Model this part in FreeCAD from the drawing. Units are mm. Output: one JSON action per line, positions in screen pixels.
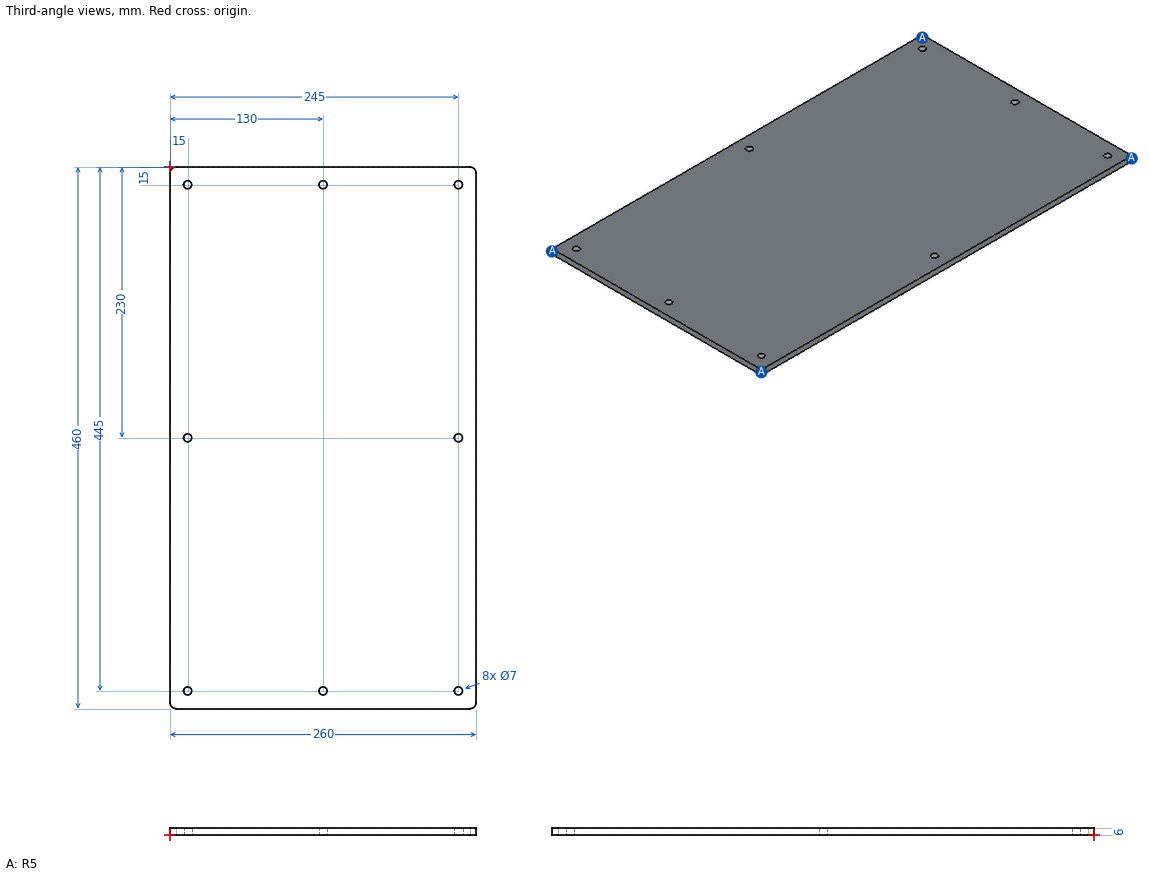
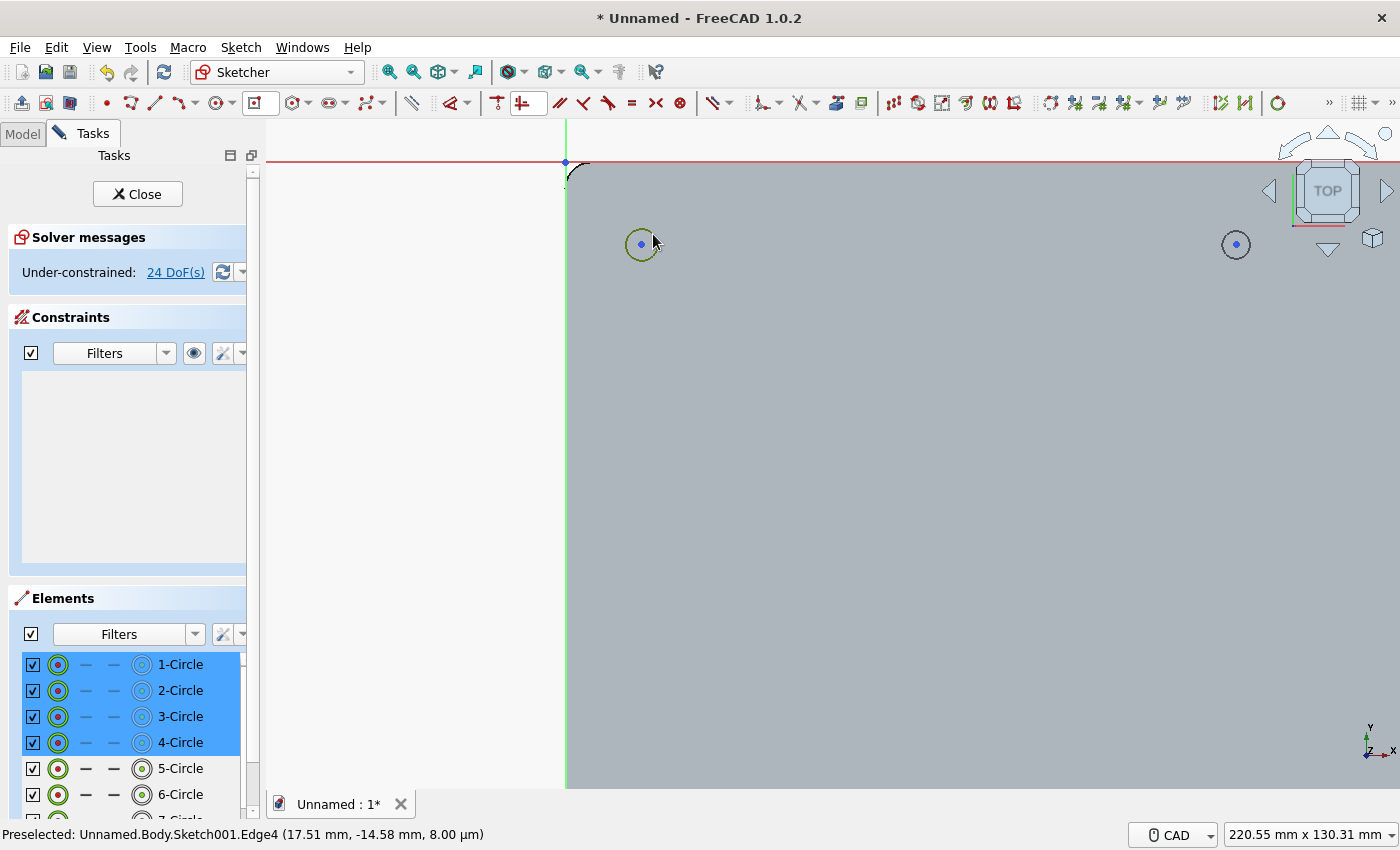
{"action": "scroll", "coordinate": [653, 236], "scroll_direction": "down", "scroll_amount": 8}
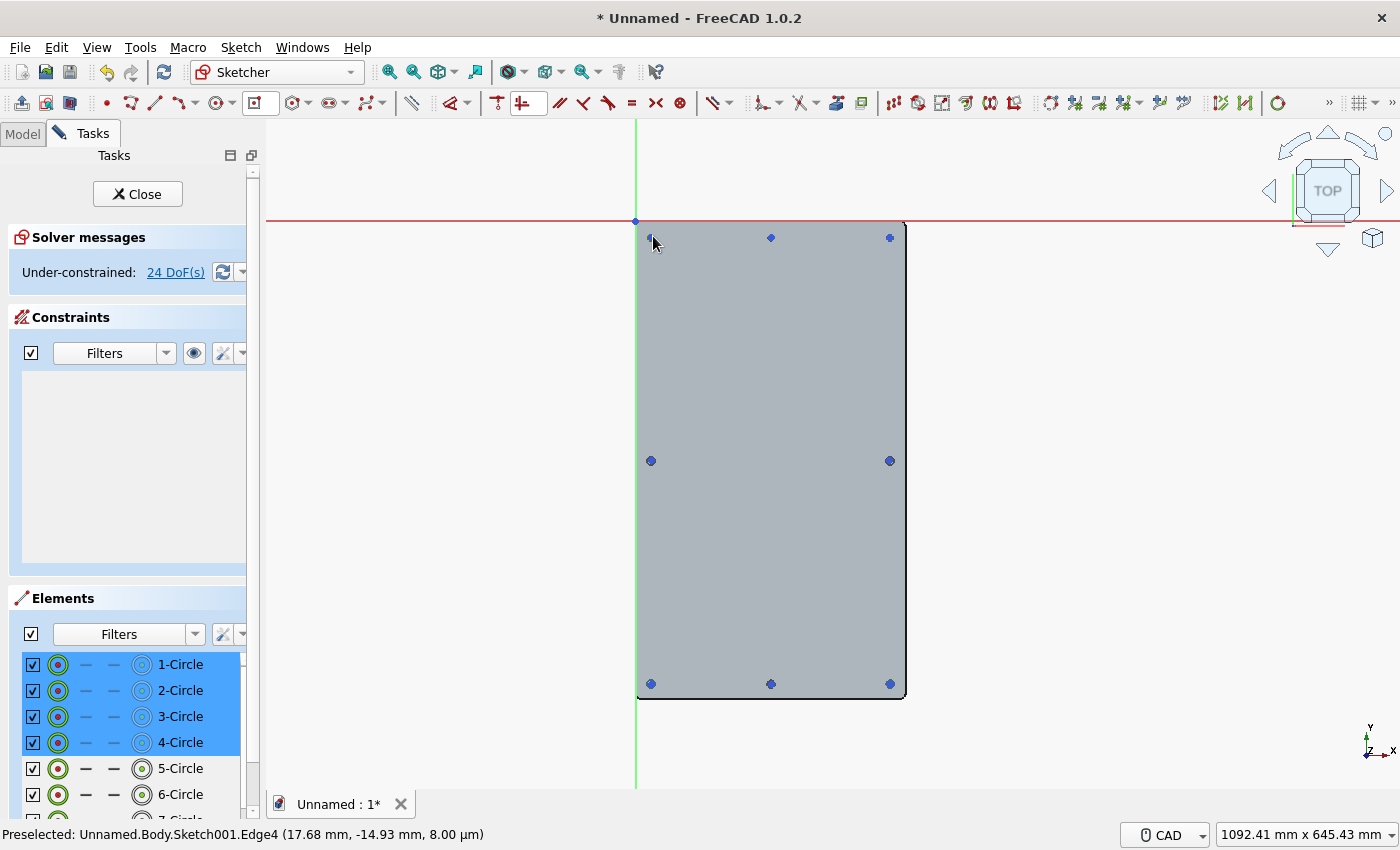
{"action": "scroll", "coordinate": [774, 681], "scroll_direction": "up", "scroll_amount": 7}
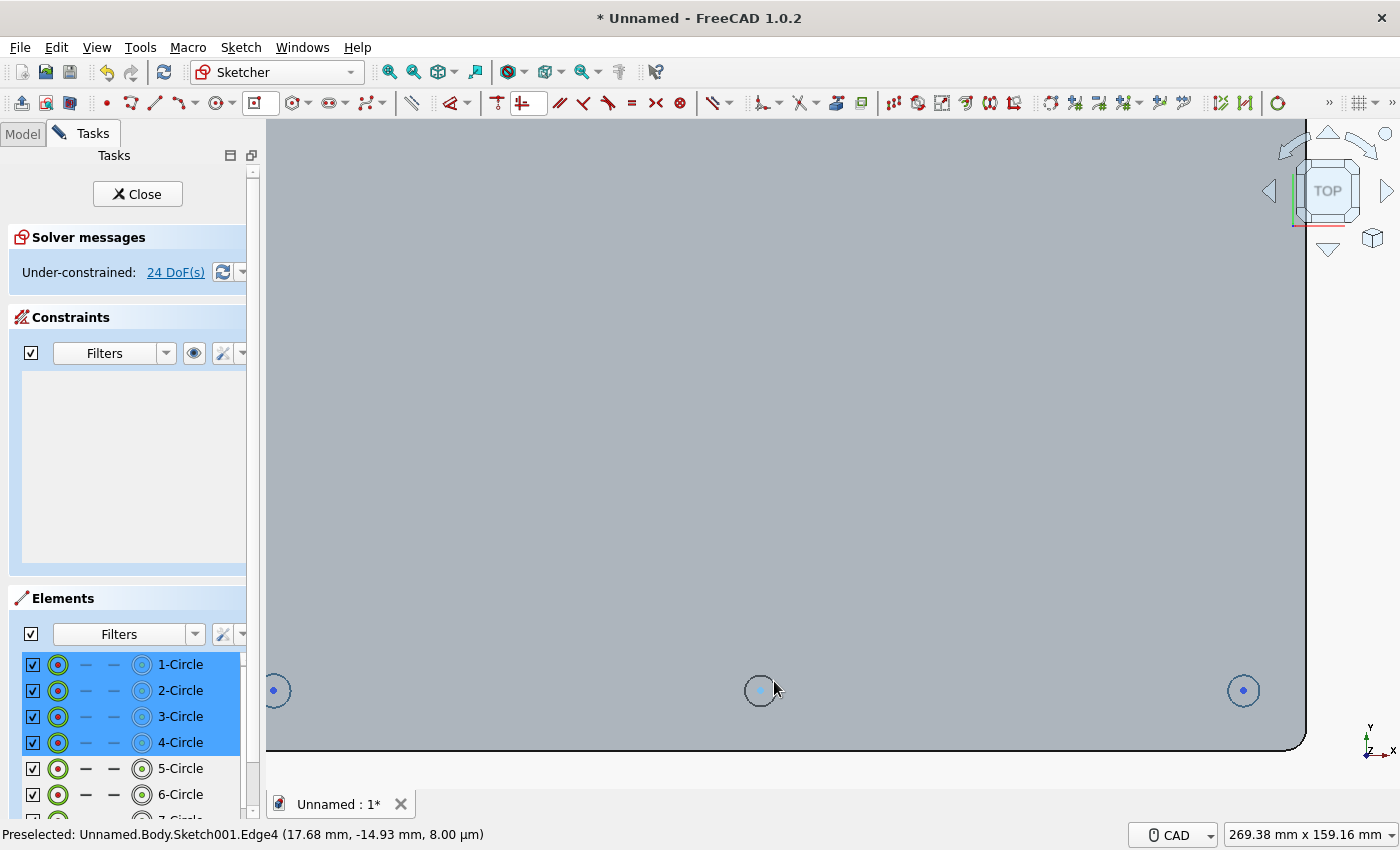
{"action": "left_click", "coordinate": [771, 680]}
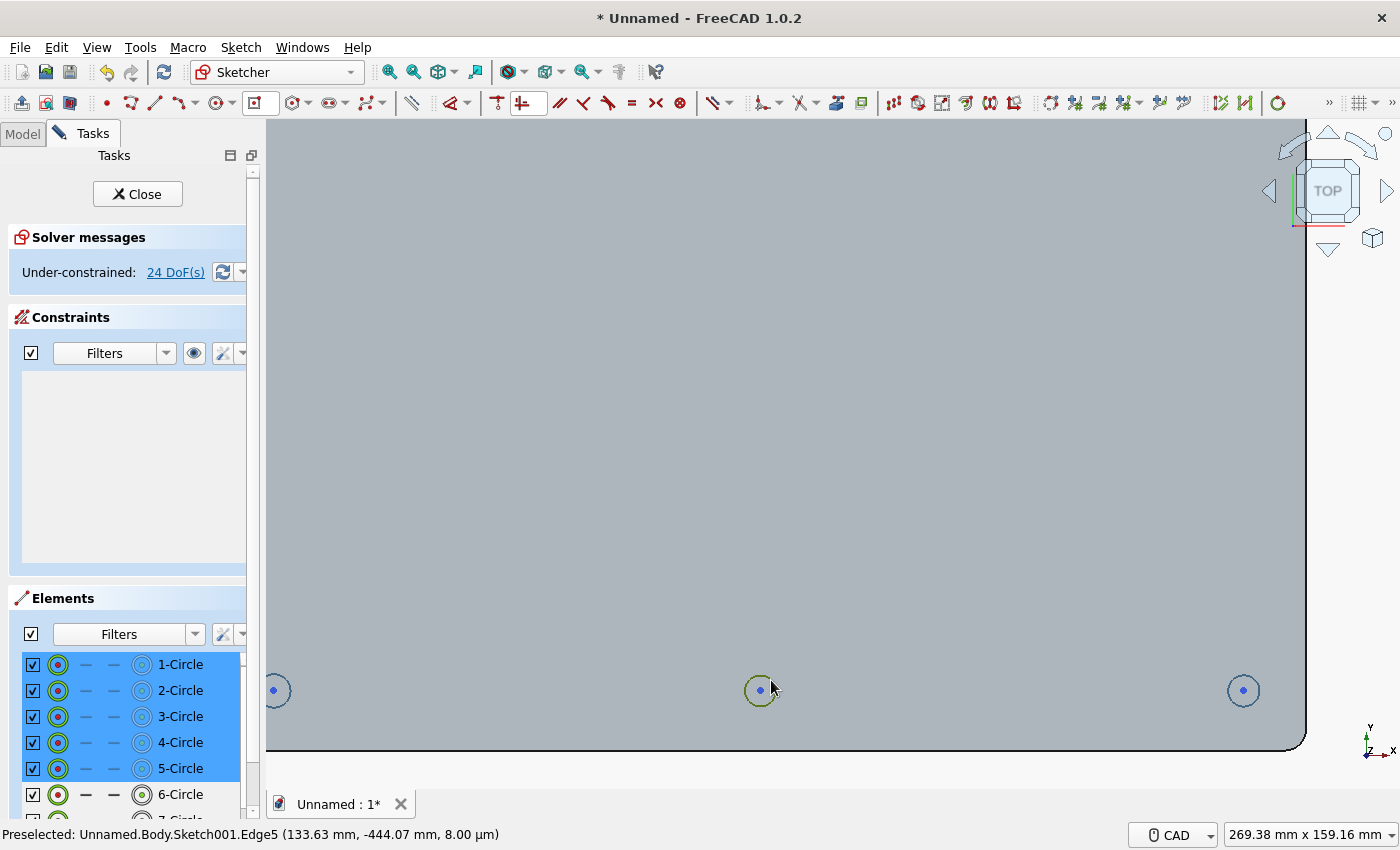
{"action": "scroll", "coordinate": [774, 682], "scroll_direction": "down", "scroll_amount": 7}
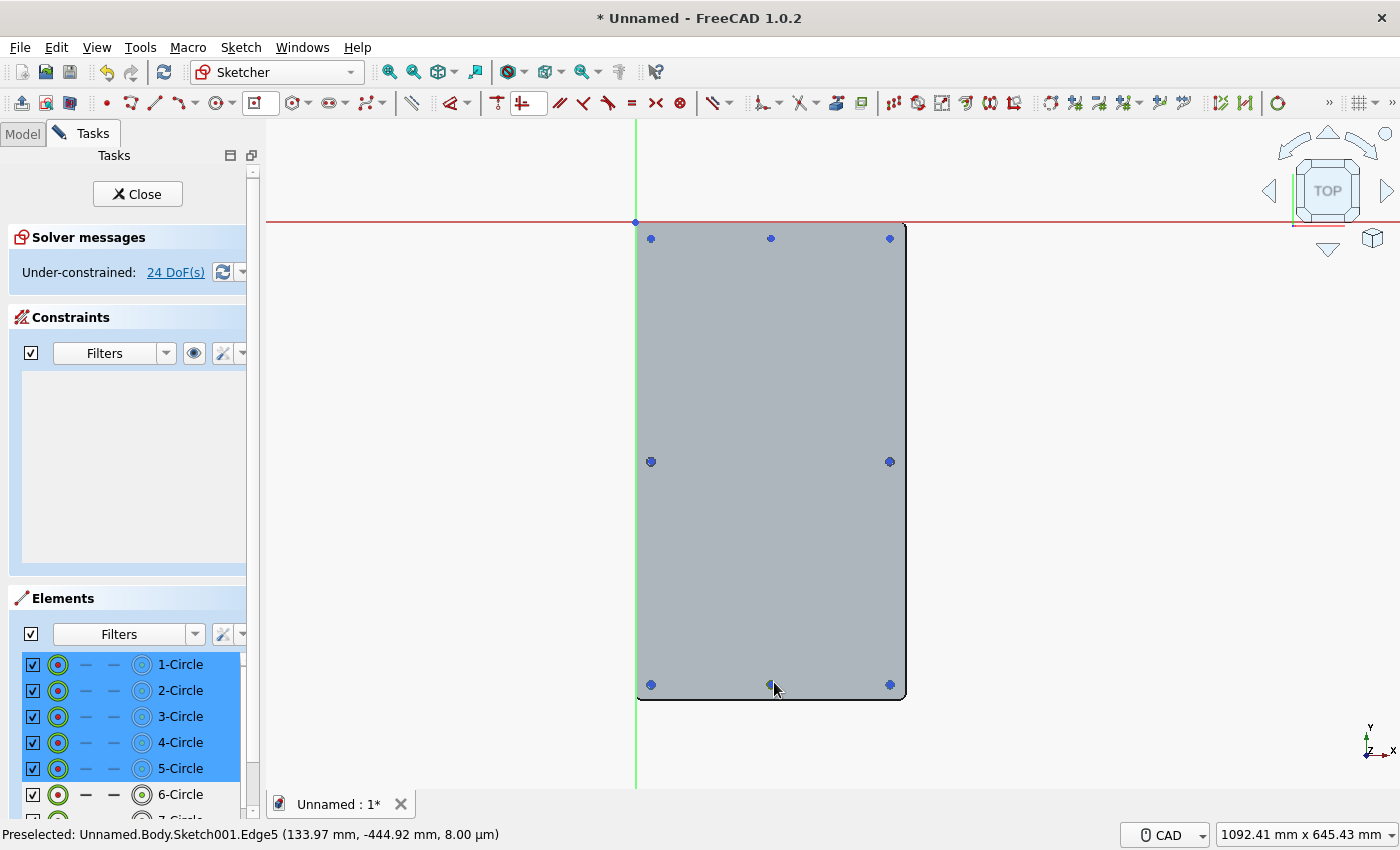
{"action": "scroll", "coordinate": [893, 459], "scroll_direction": "up", "scroll_amount": 7}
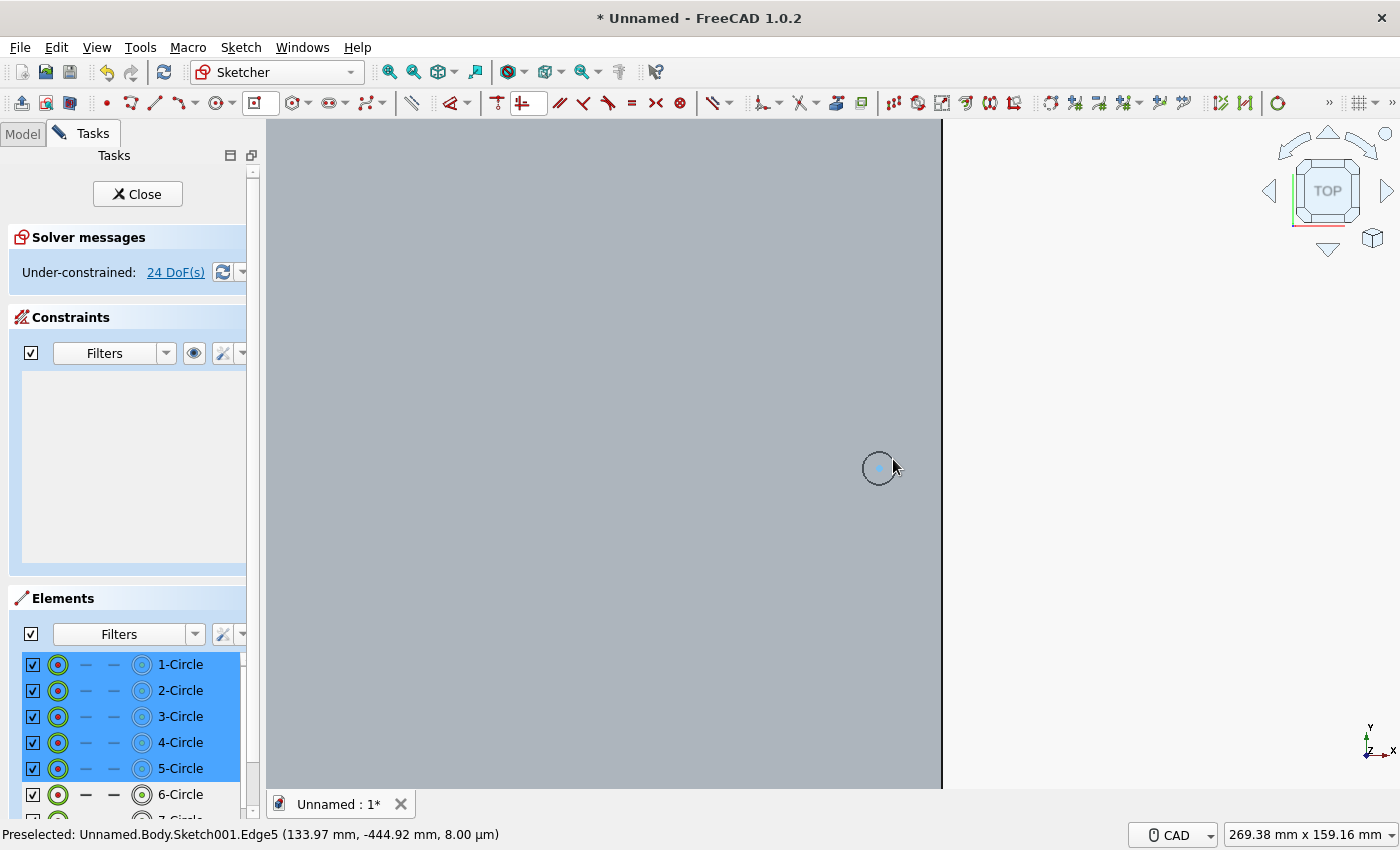
{"action": "left_click", "coordinate": [891, 457]}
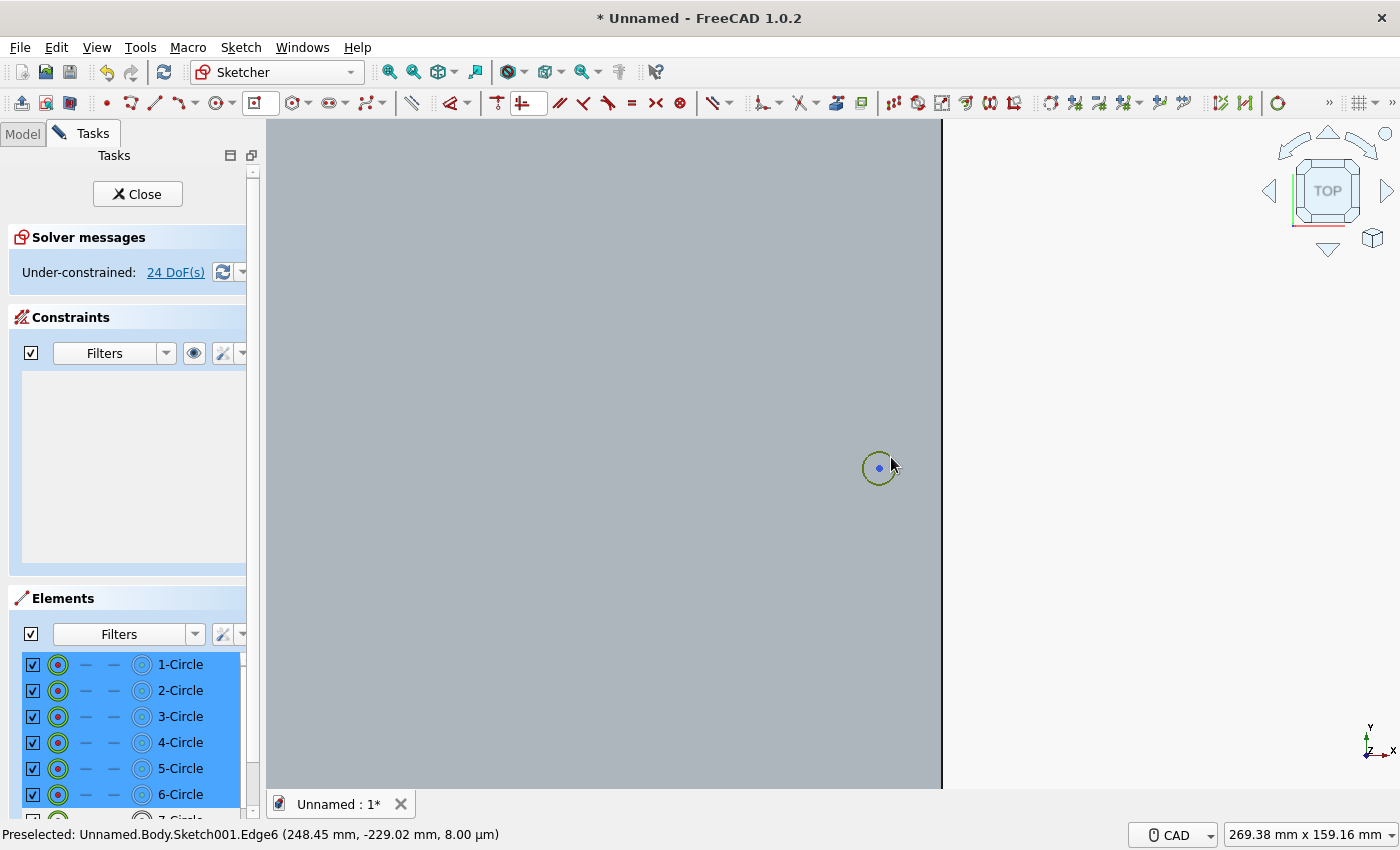
{"action": "scroll", "coordinate": [893, 458], "scroll_direction": "down", "scroll_amount": 7}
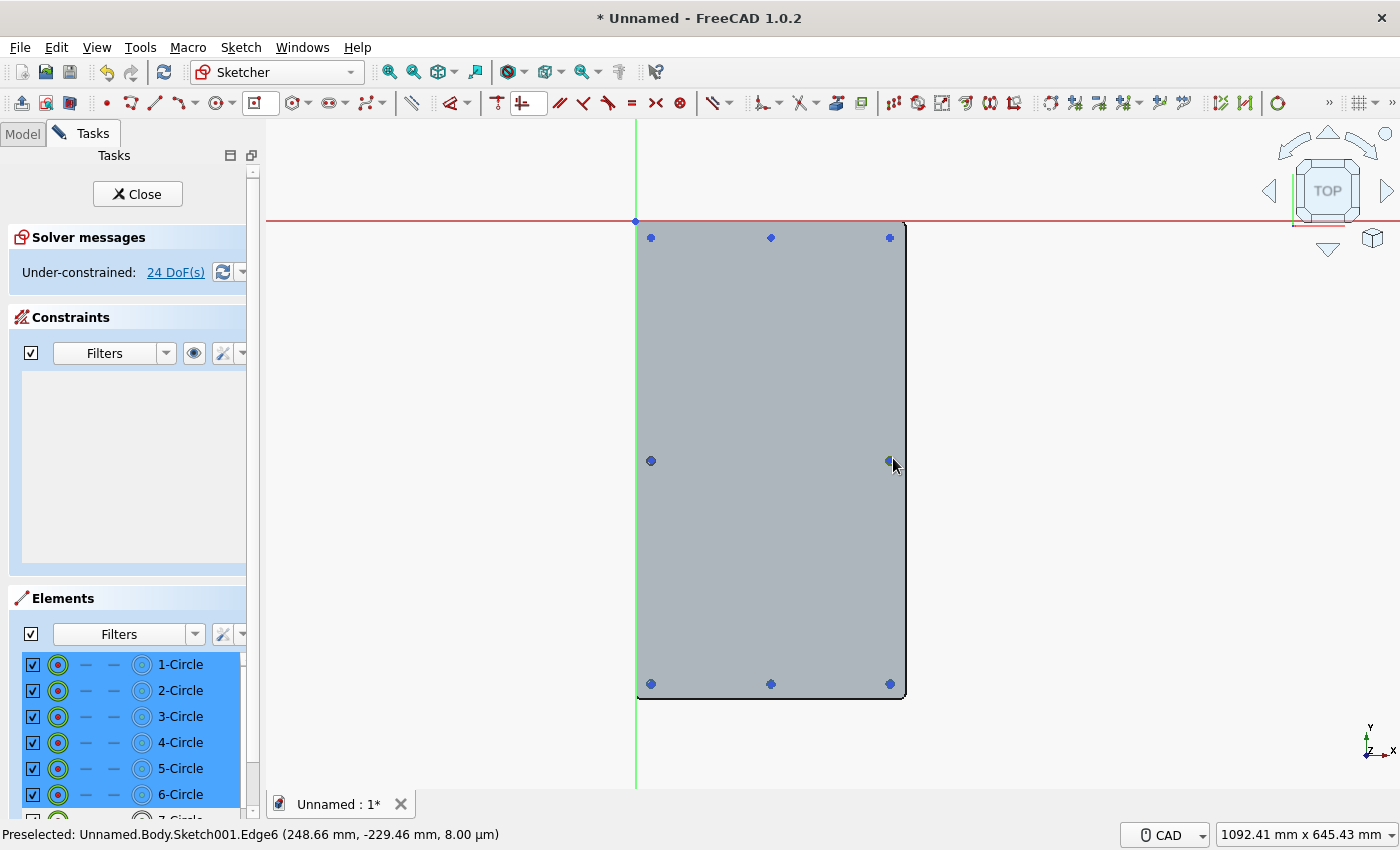
{"action": "scroll", "coordinate": [773, 236], "scroll_direction": "up", "scroll_amount": 9}